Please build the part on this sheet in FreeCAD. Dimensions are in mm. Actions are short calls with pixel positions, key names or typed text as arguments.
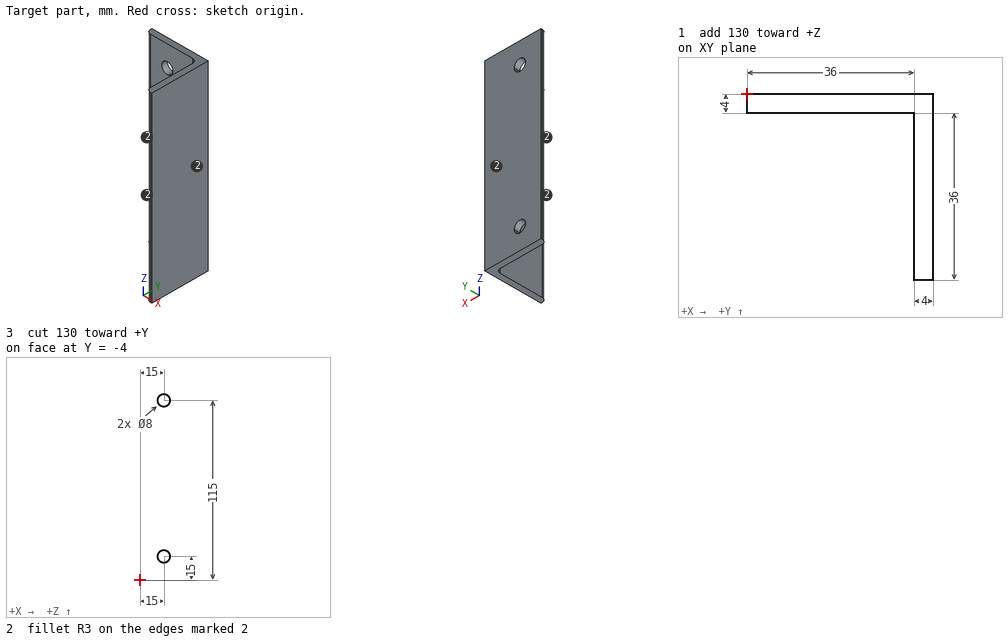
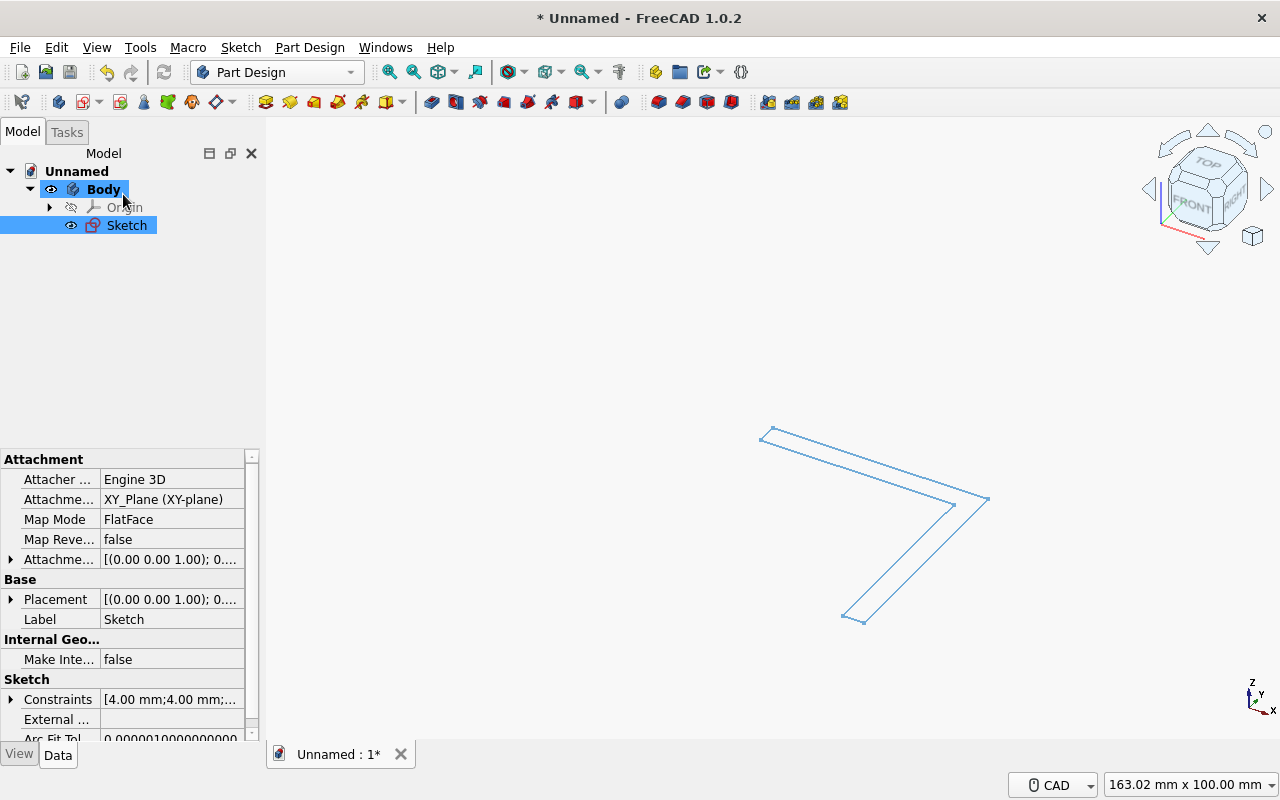
click(266, 102)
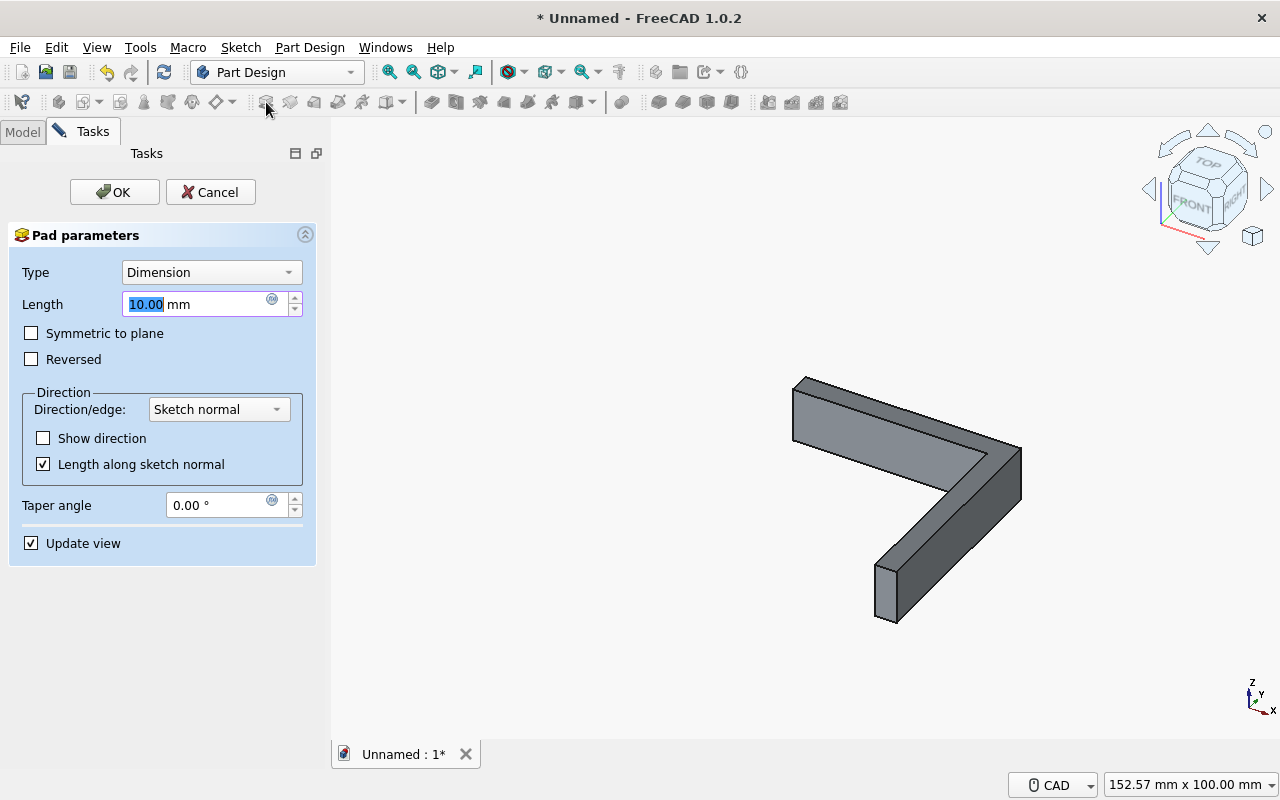
text(130)
key(Tab)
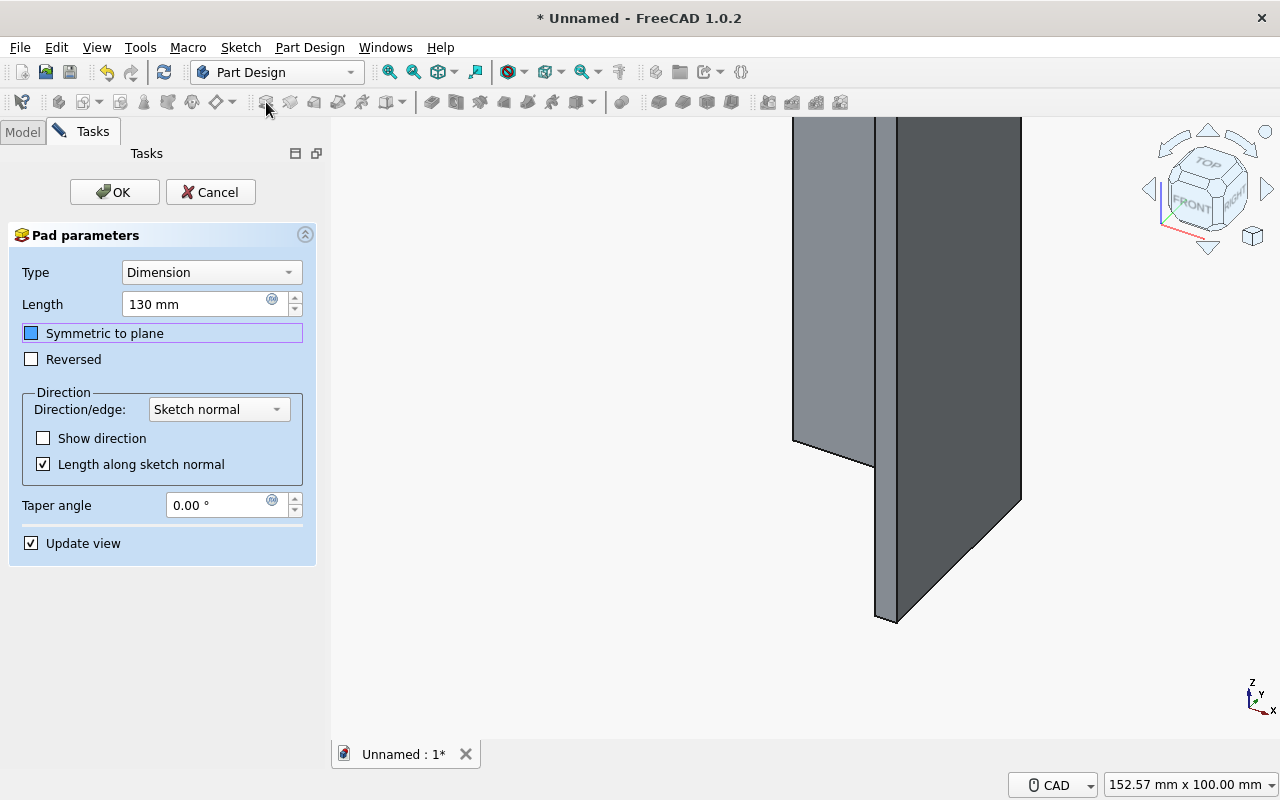
click(115, 192)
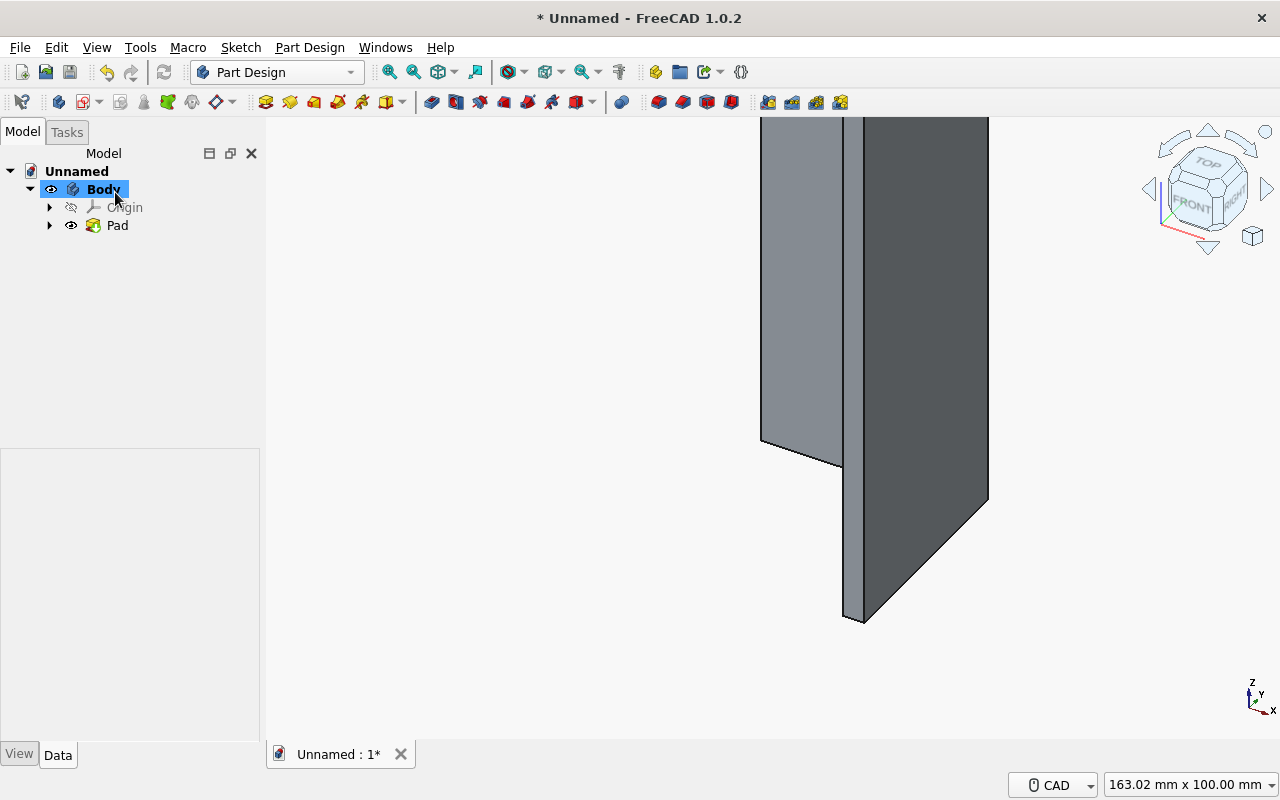
click(390, 72)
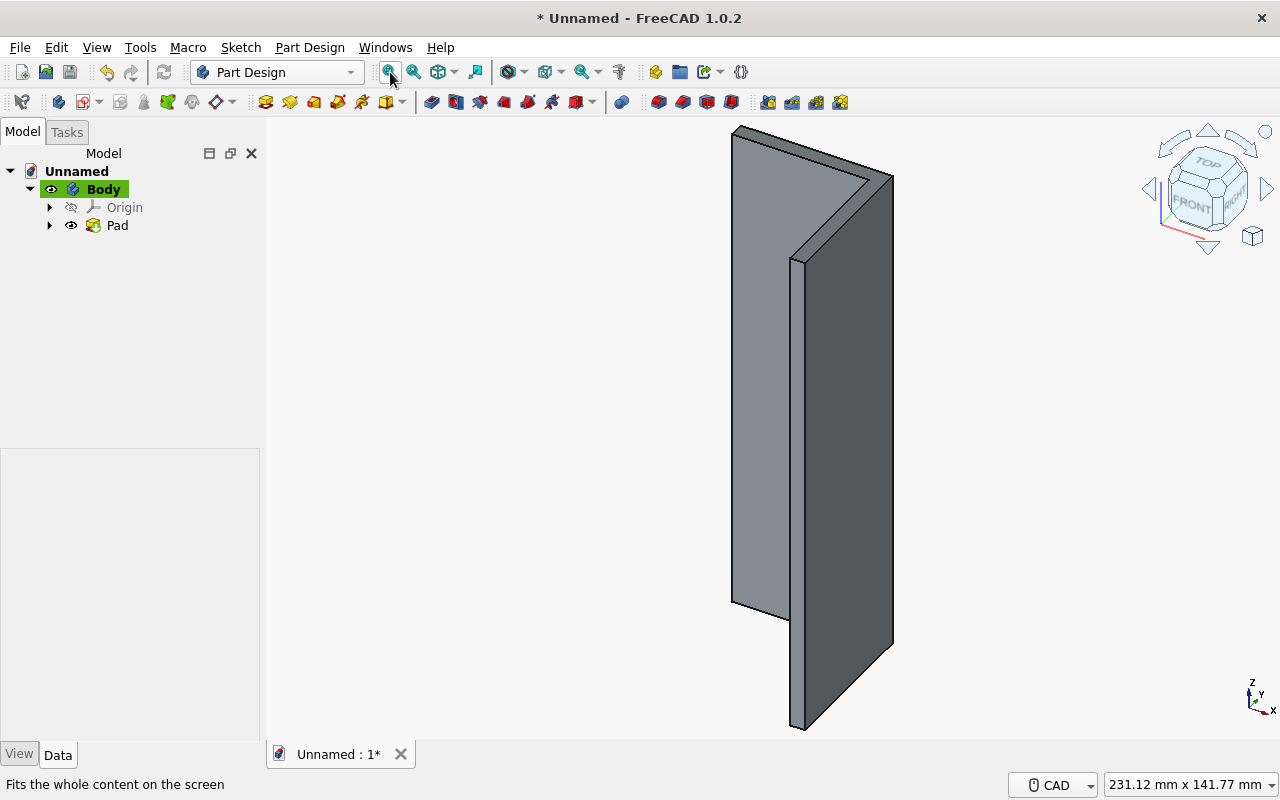
key(0)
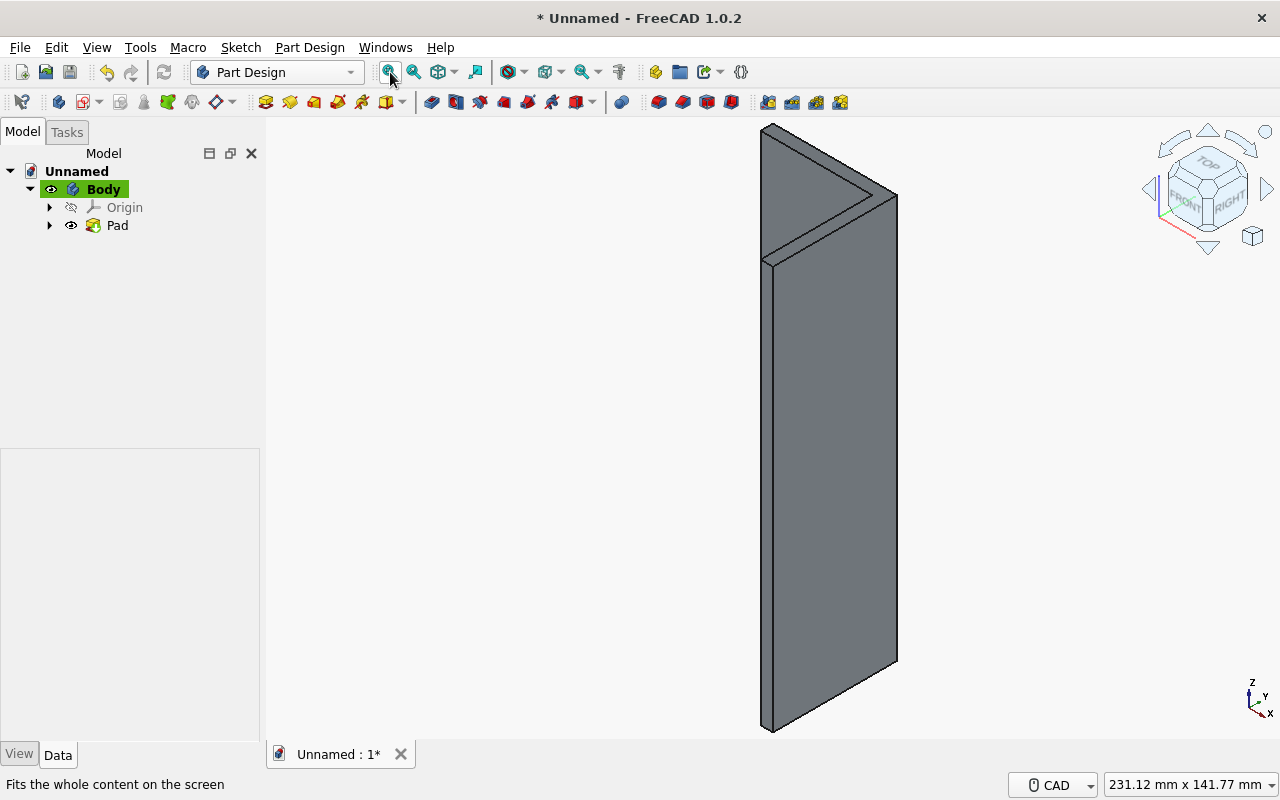
key(2)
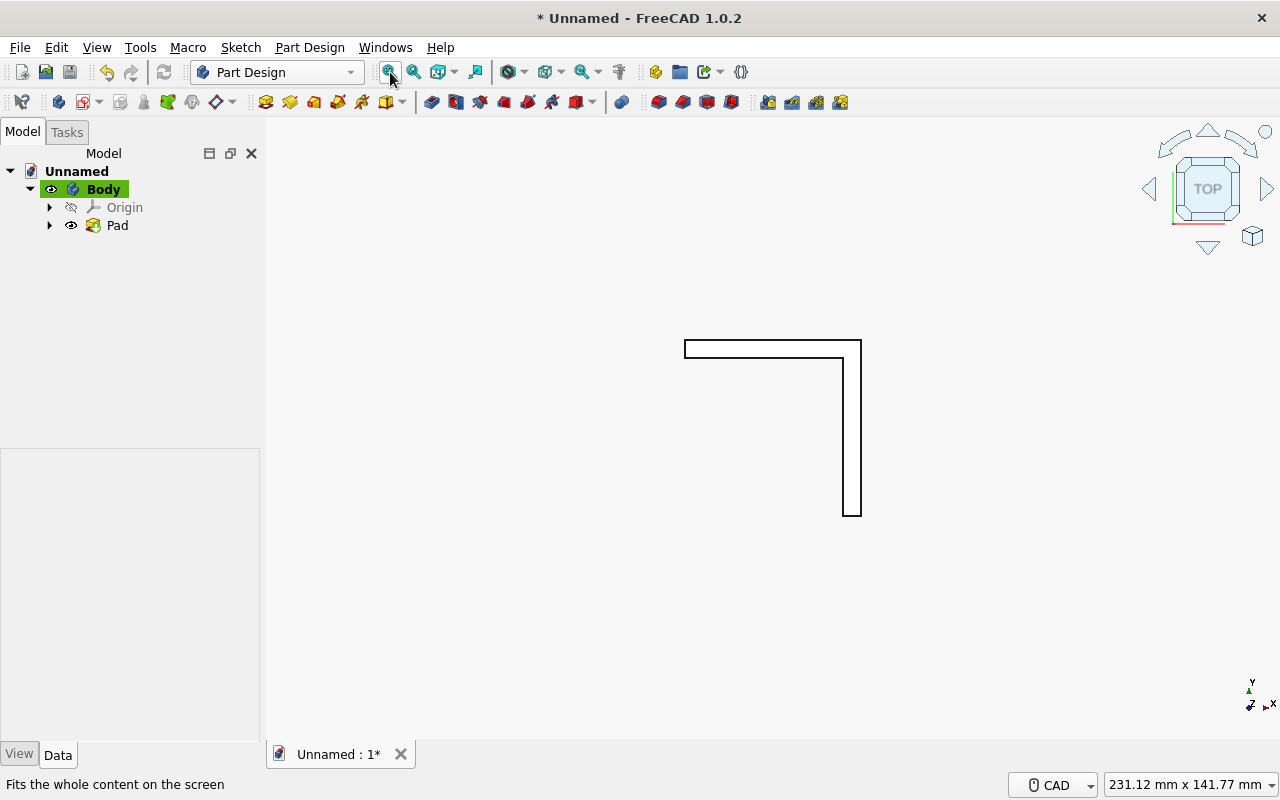
click(390, 72)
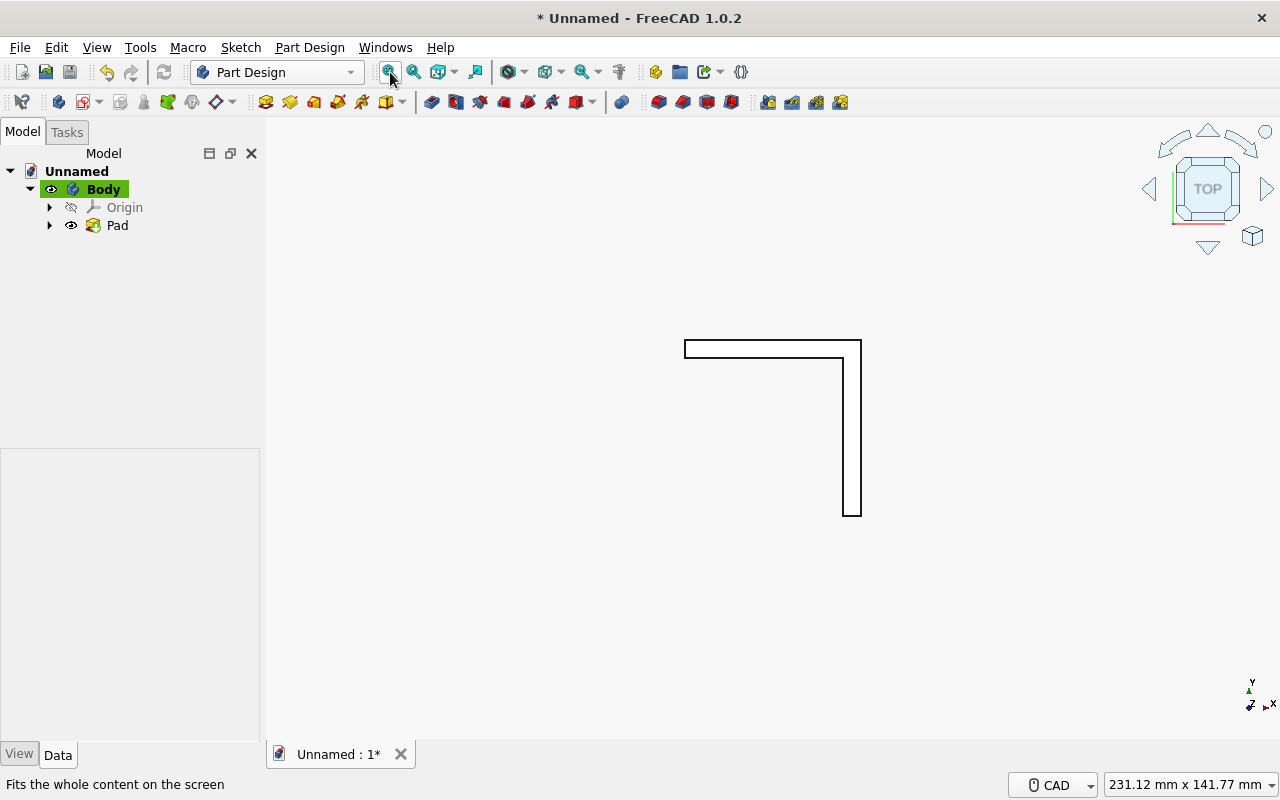
key(1)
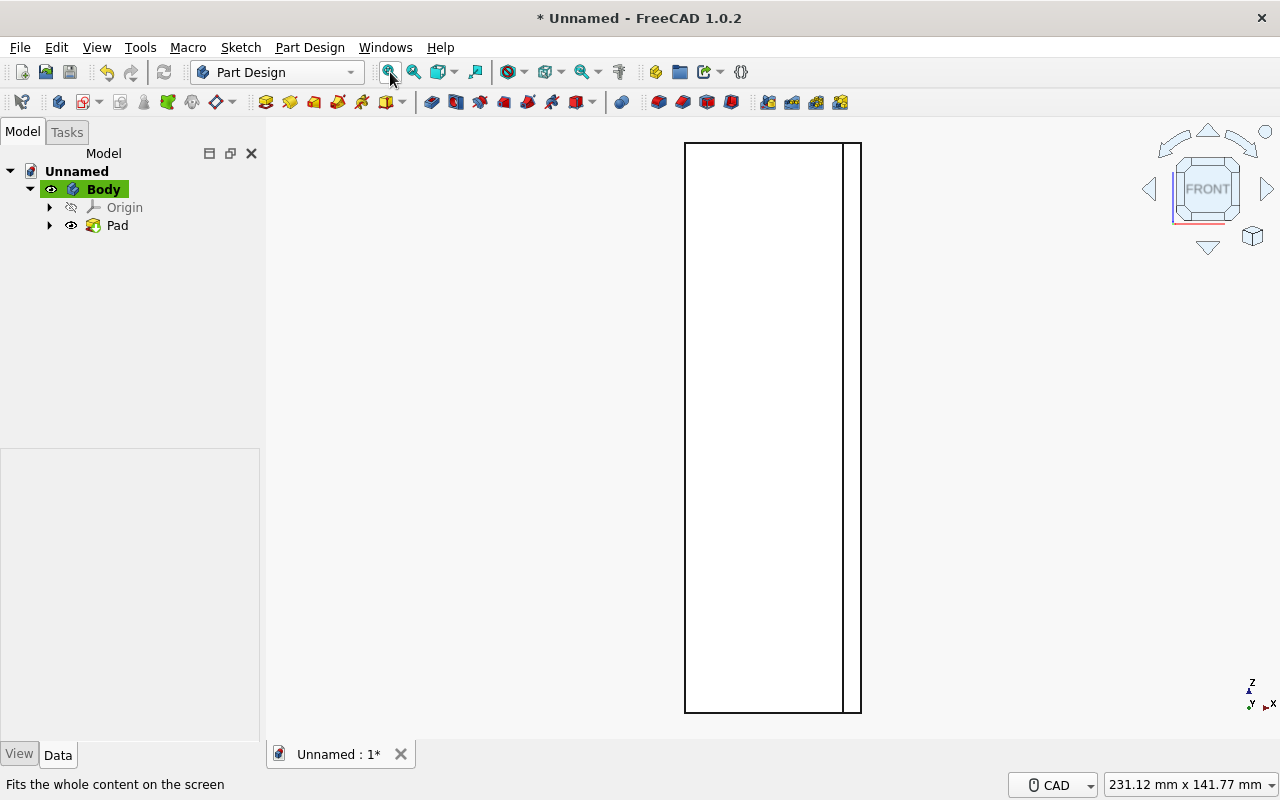
click(685, 427)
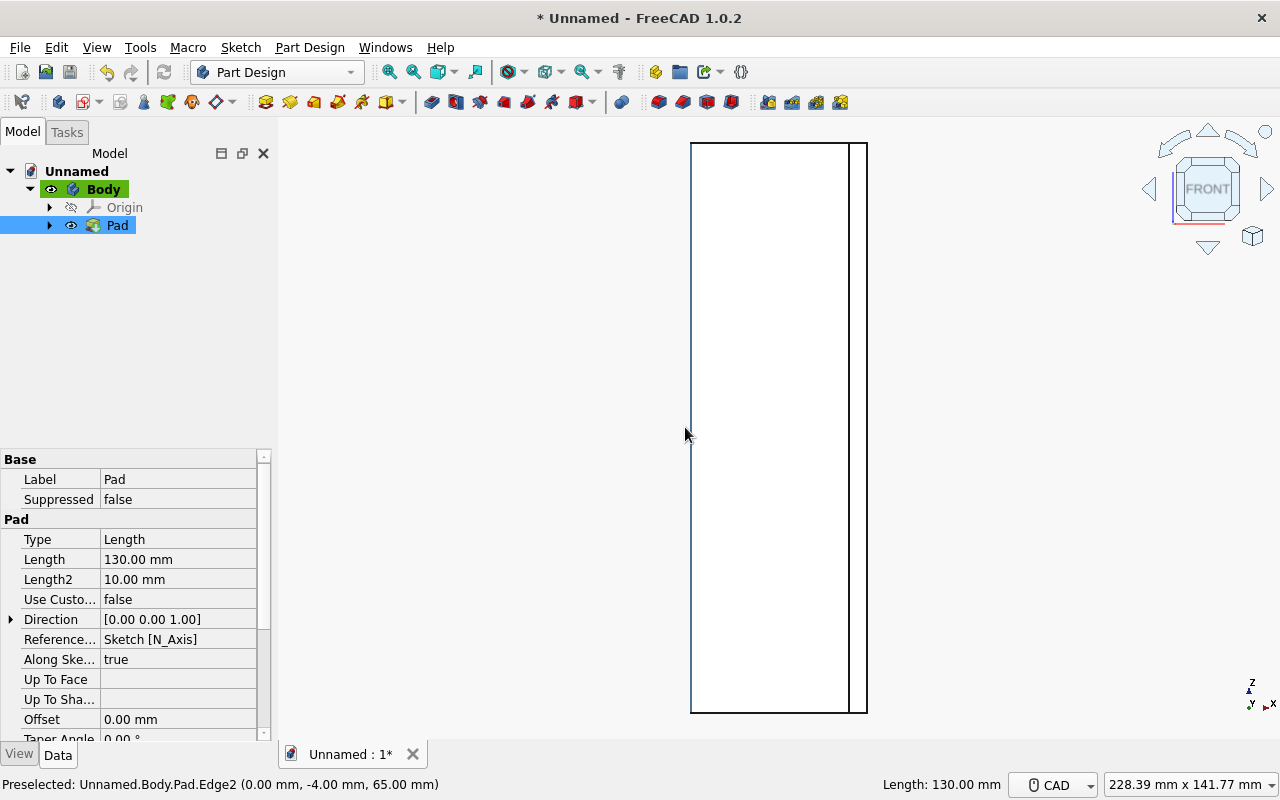
click(849, 427, ctrl)